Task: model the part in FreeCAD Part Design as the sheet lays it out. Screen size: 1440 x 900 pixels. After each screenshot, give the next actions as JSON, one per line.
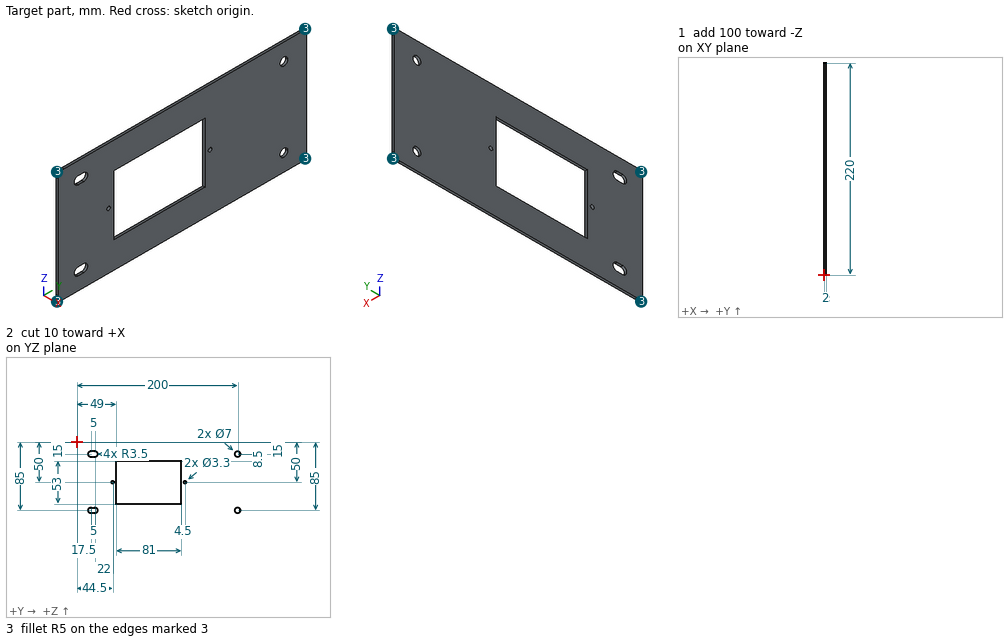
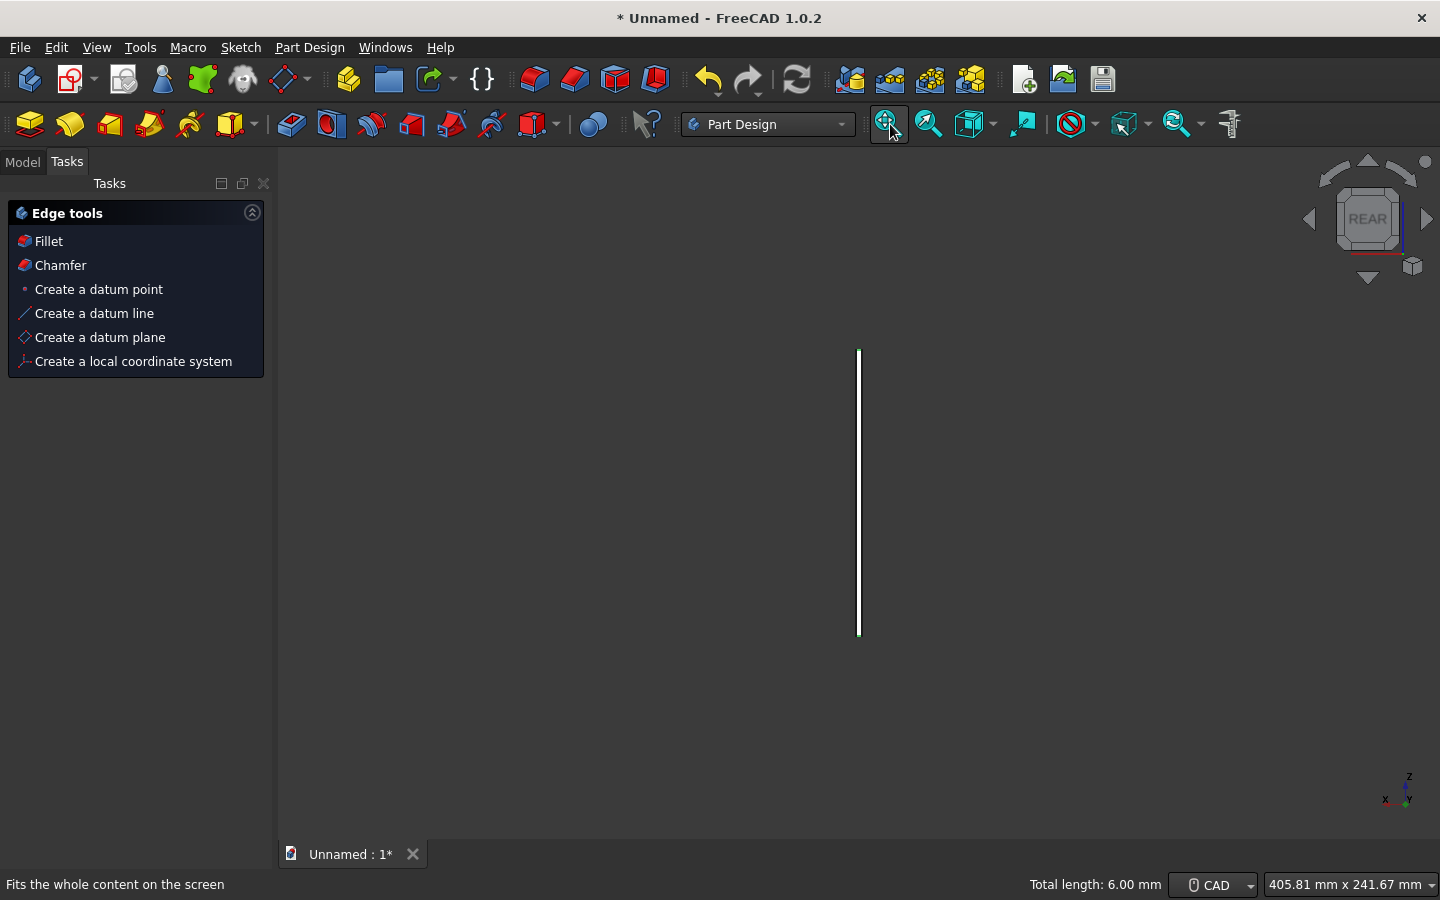
{"action": "key", "text": "6"}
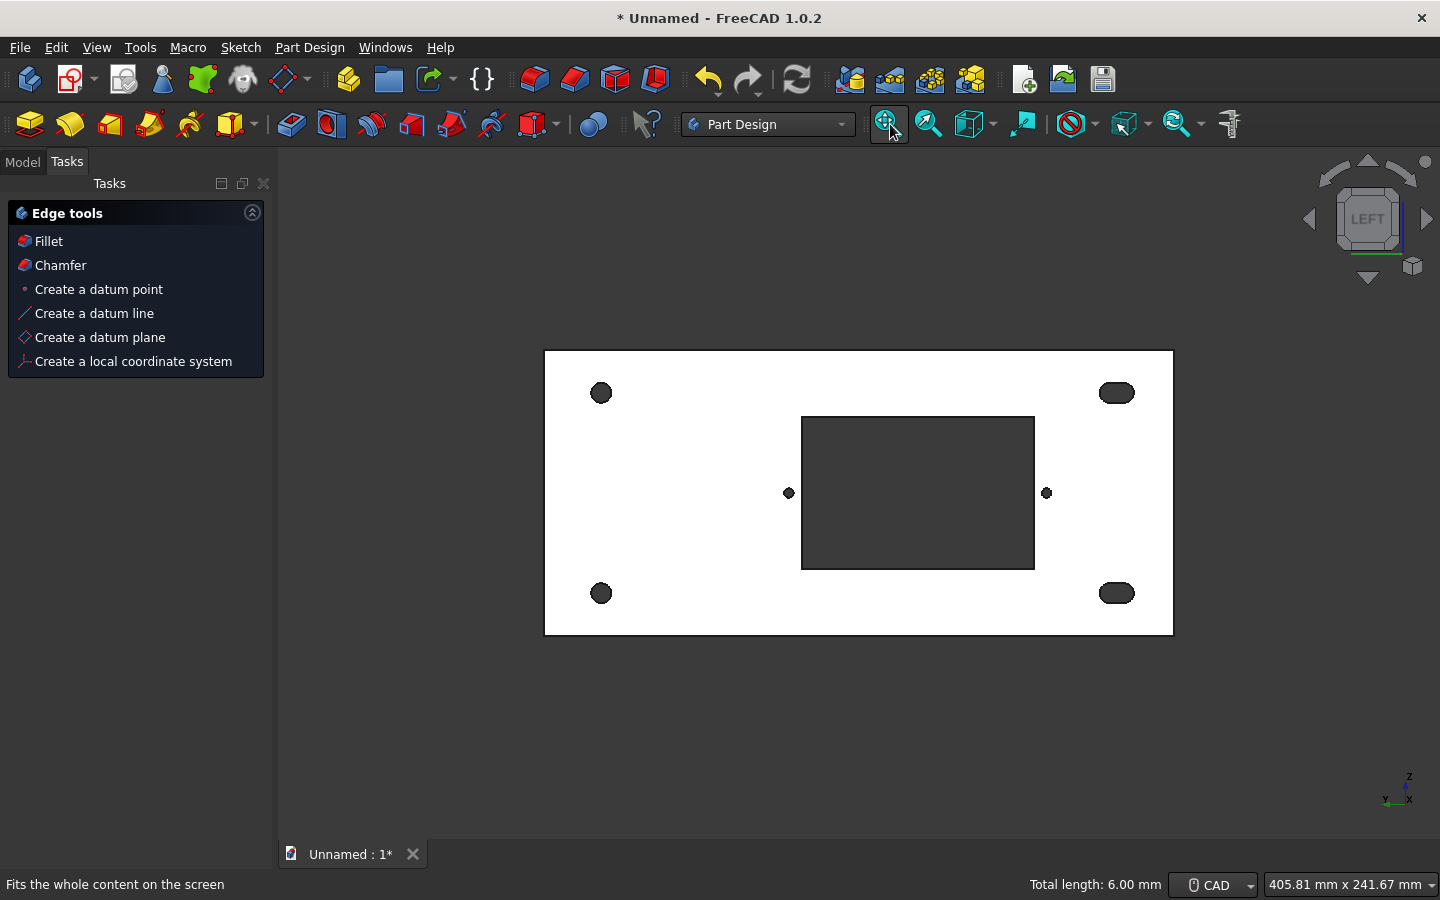
{"action": "scroll", "coordinate": [1174, 349], "scroll_direction": "up", "scroll_amount": 10}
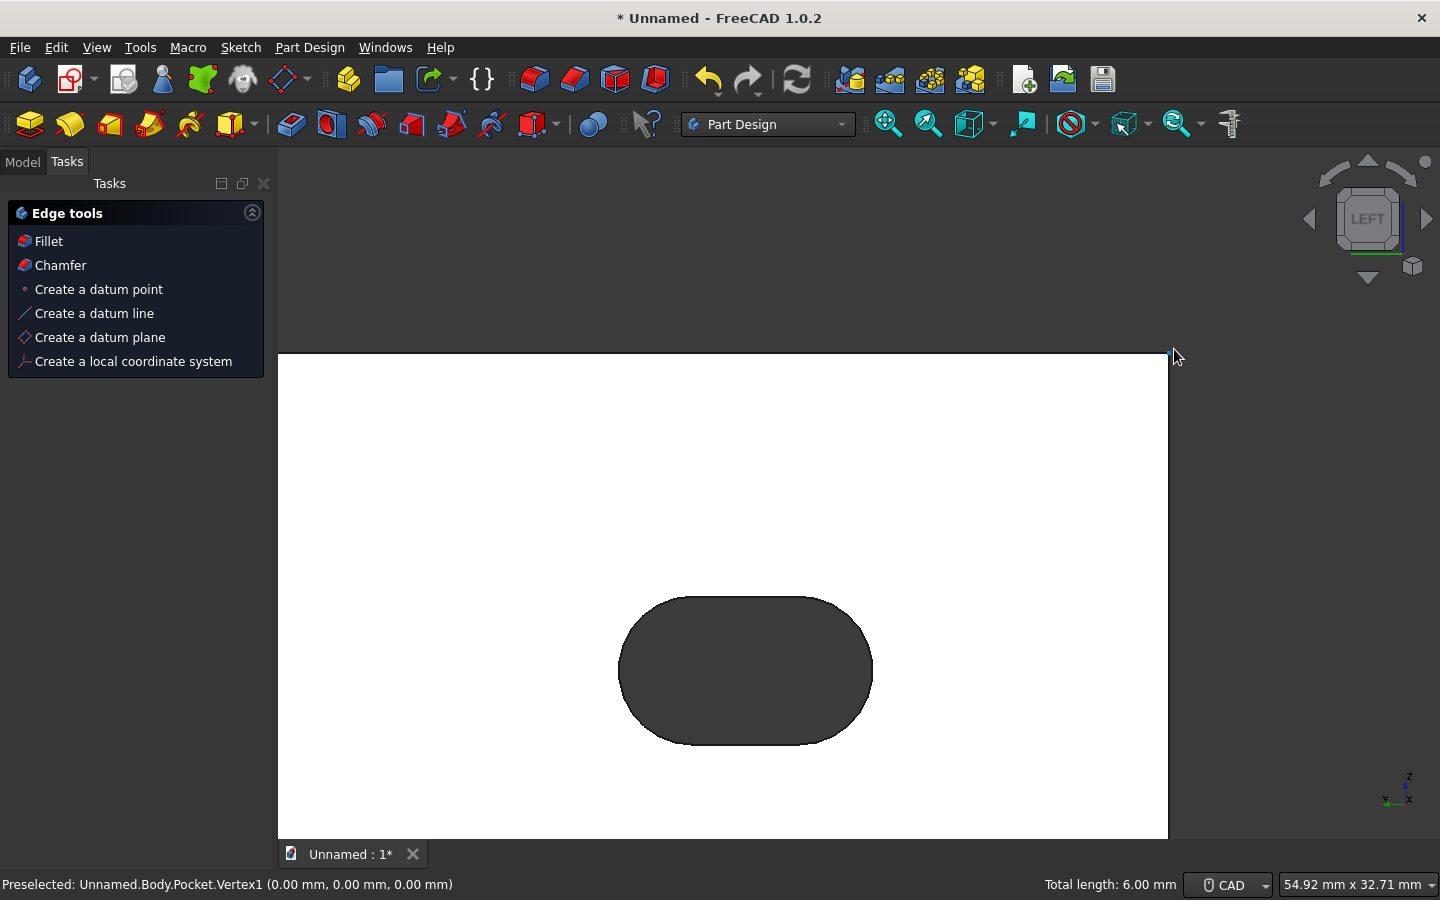
{"action": "left_click", "coordinate": [890, 124]}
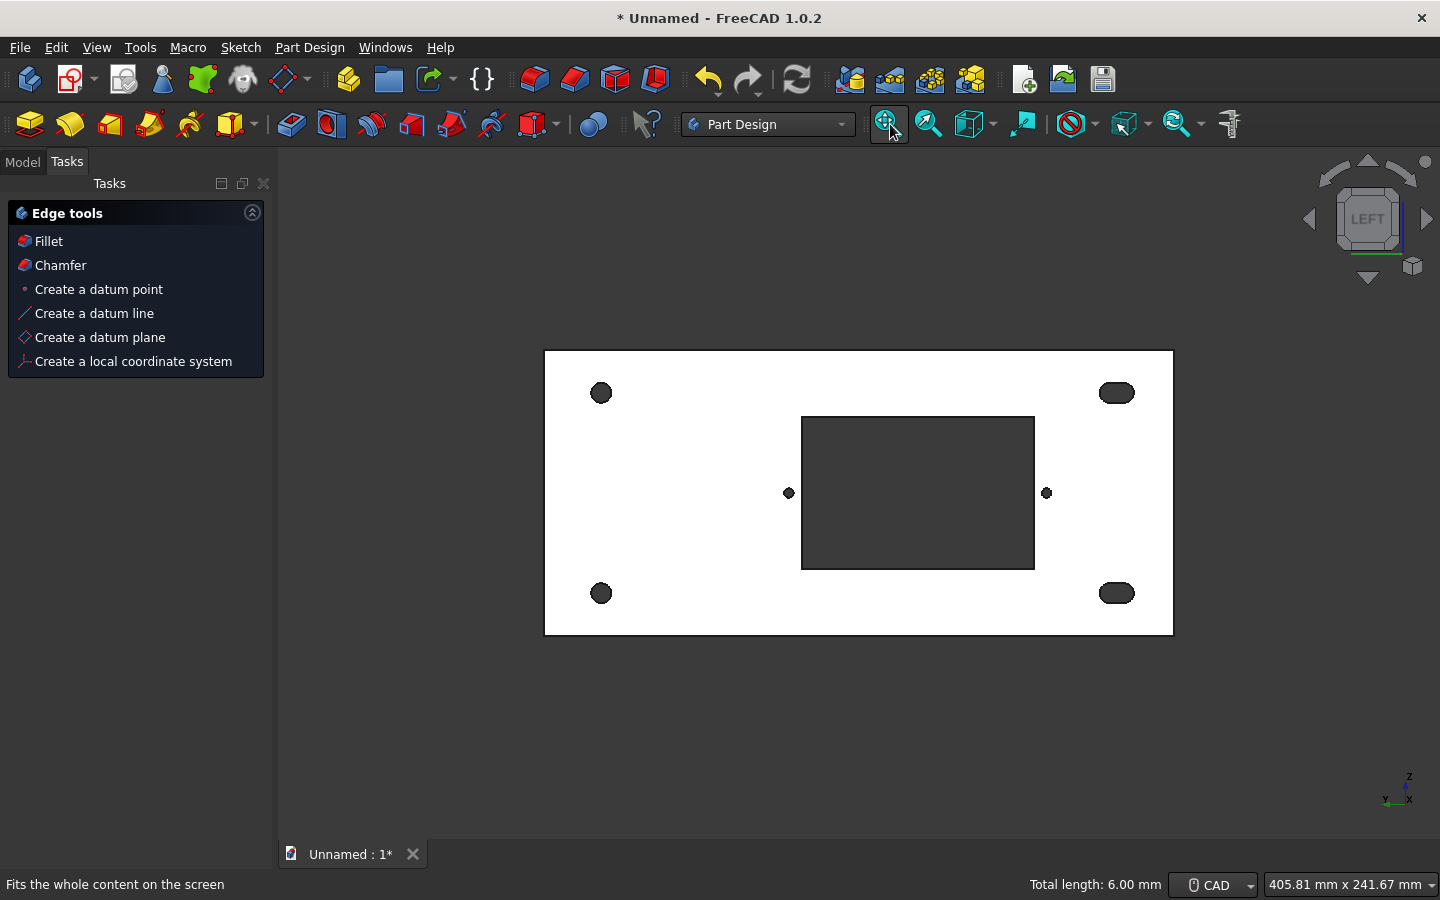
{"action": "key", "text": "v 3"}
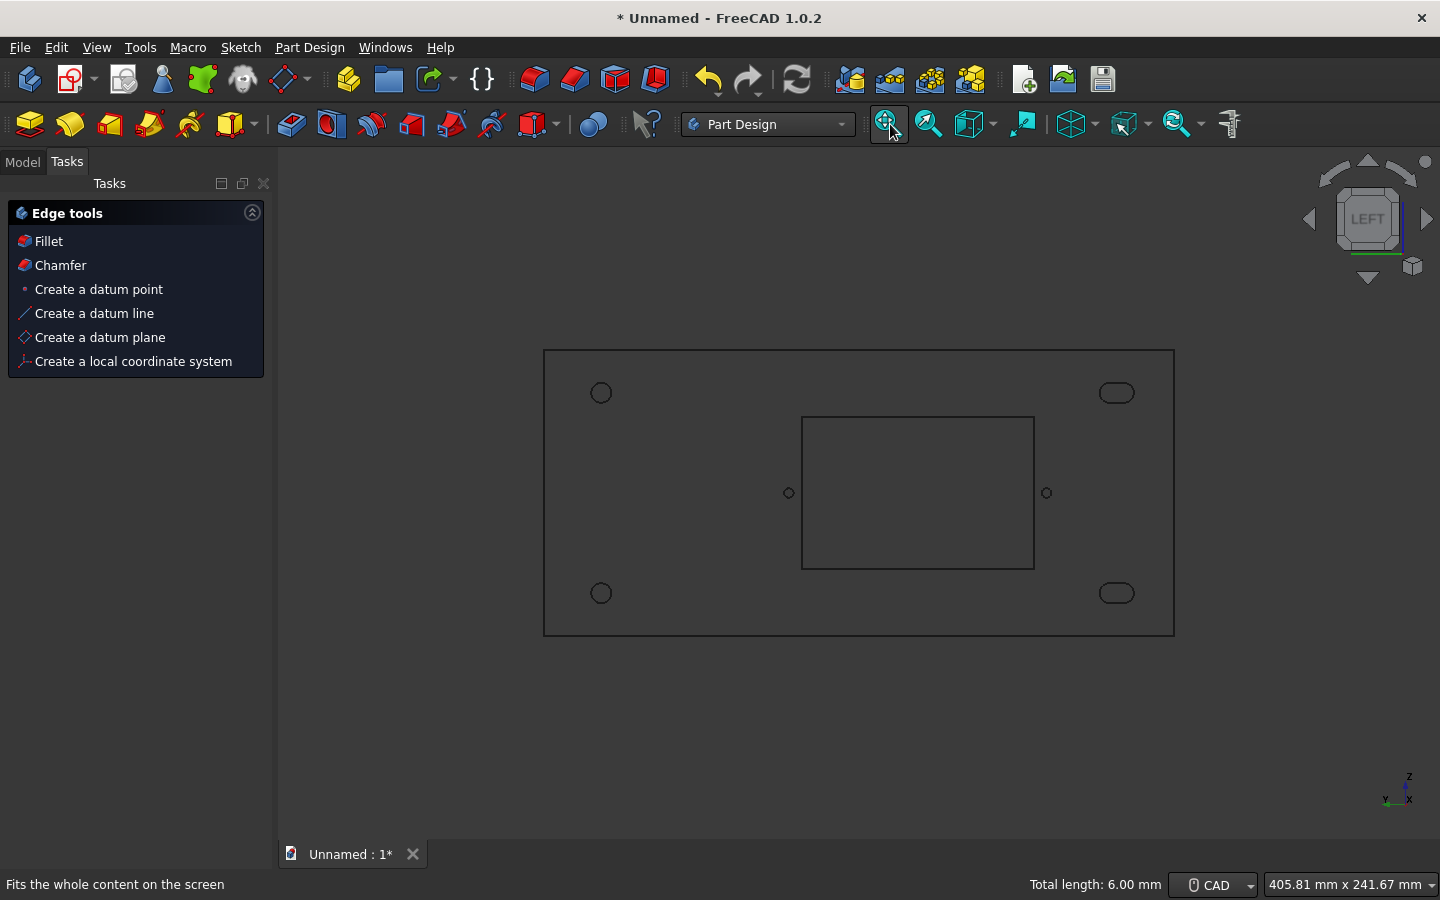
{"action": "key", "text": "0"}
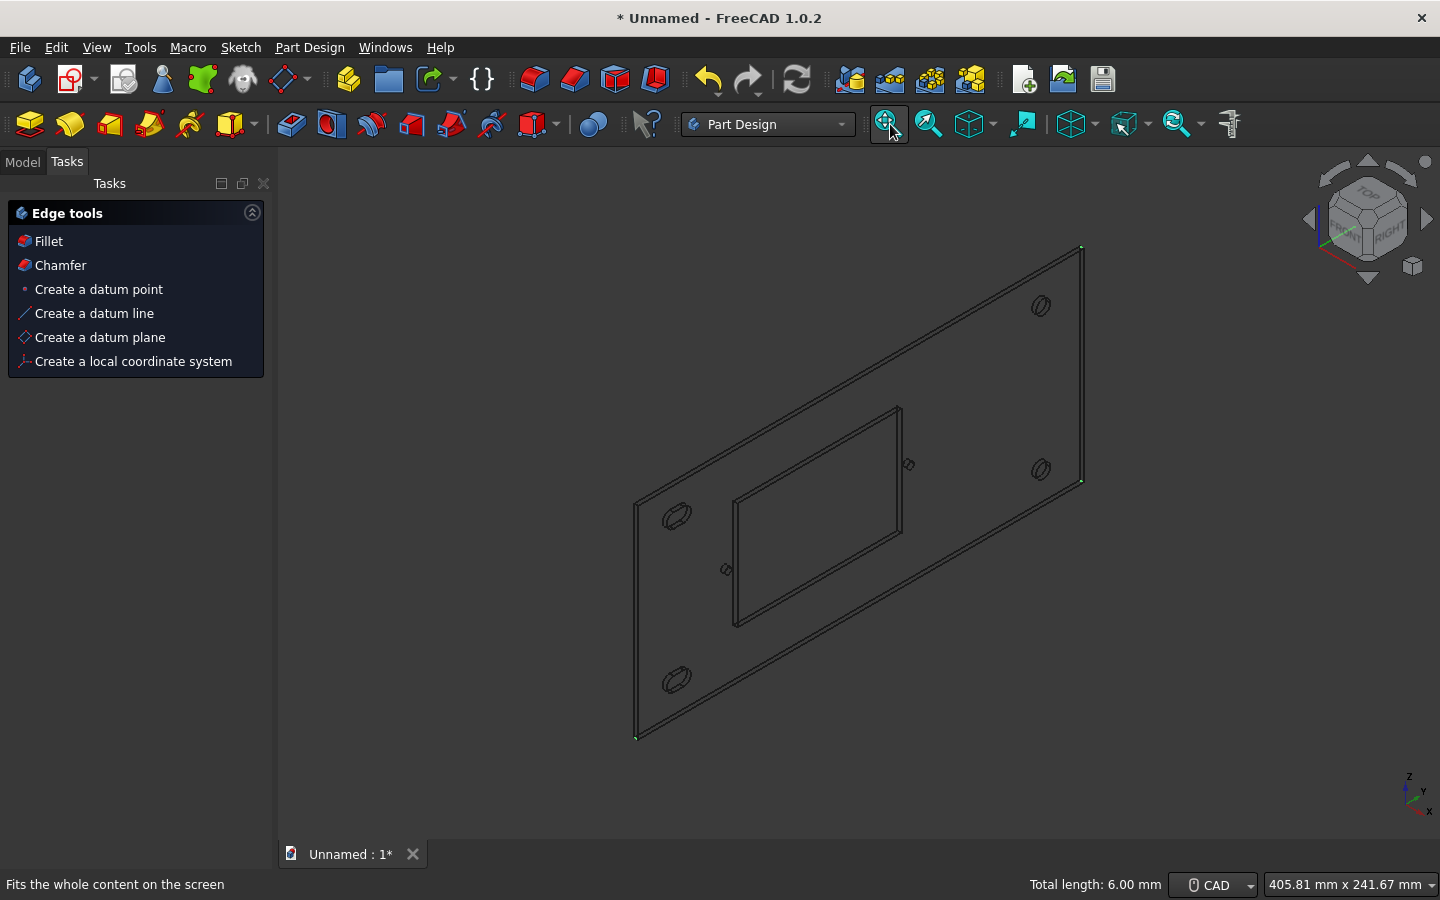
{"action": "scroll", "coordinate": [636, 504], "scroll_direction": "up", "scroll_amount": 10}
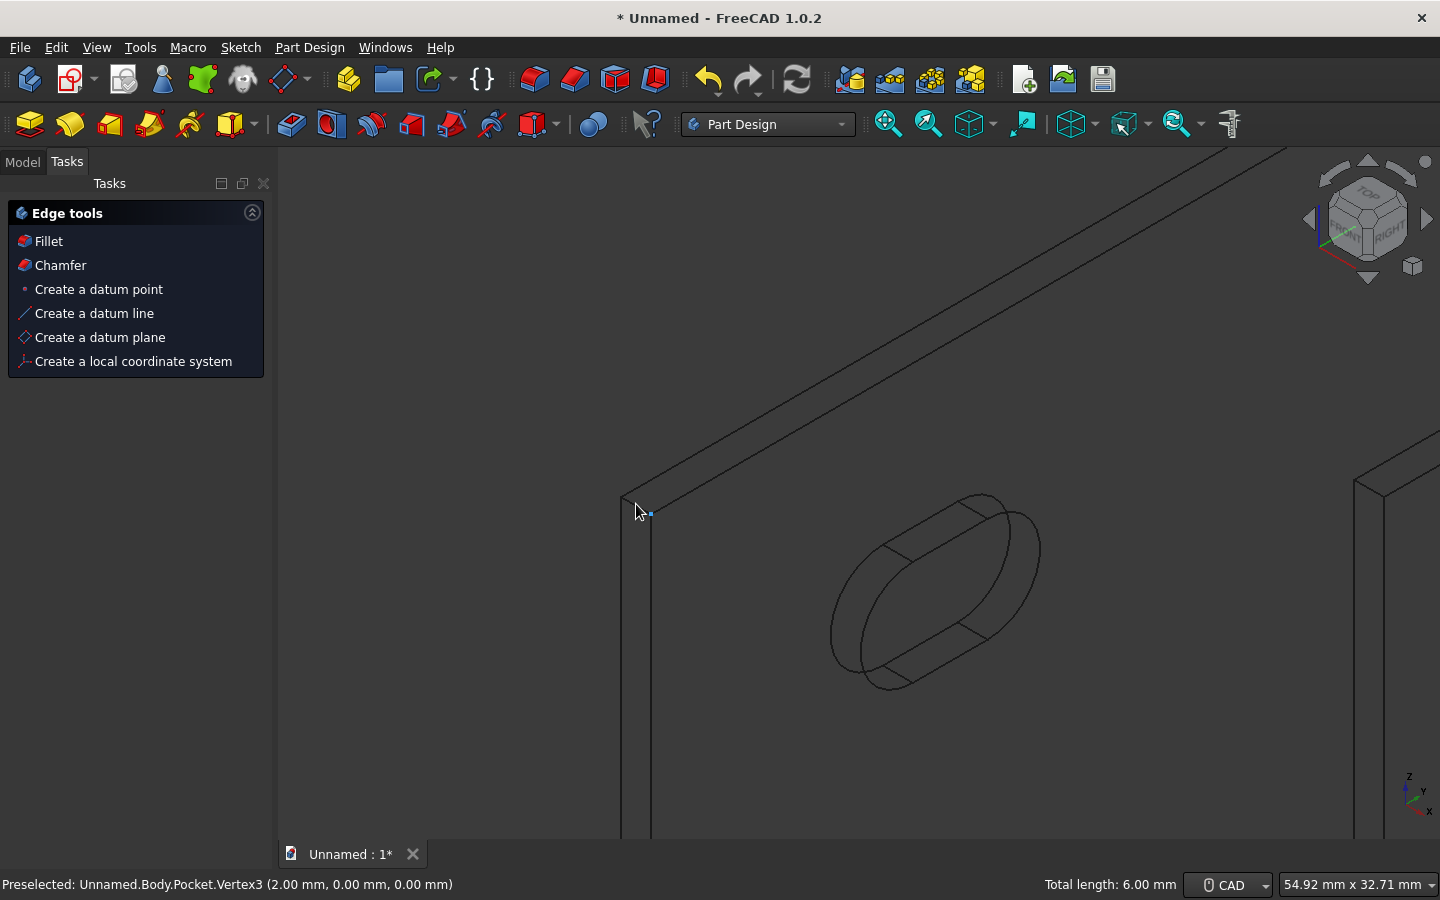
{"action": "left_click", "coordinate": [636, 505], "text": "ctrl"}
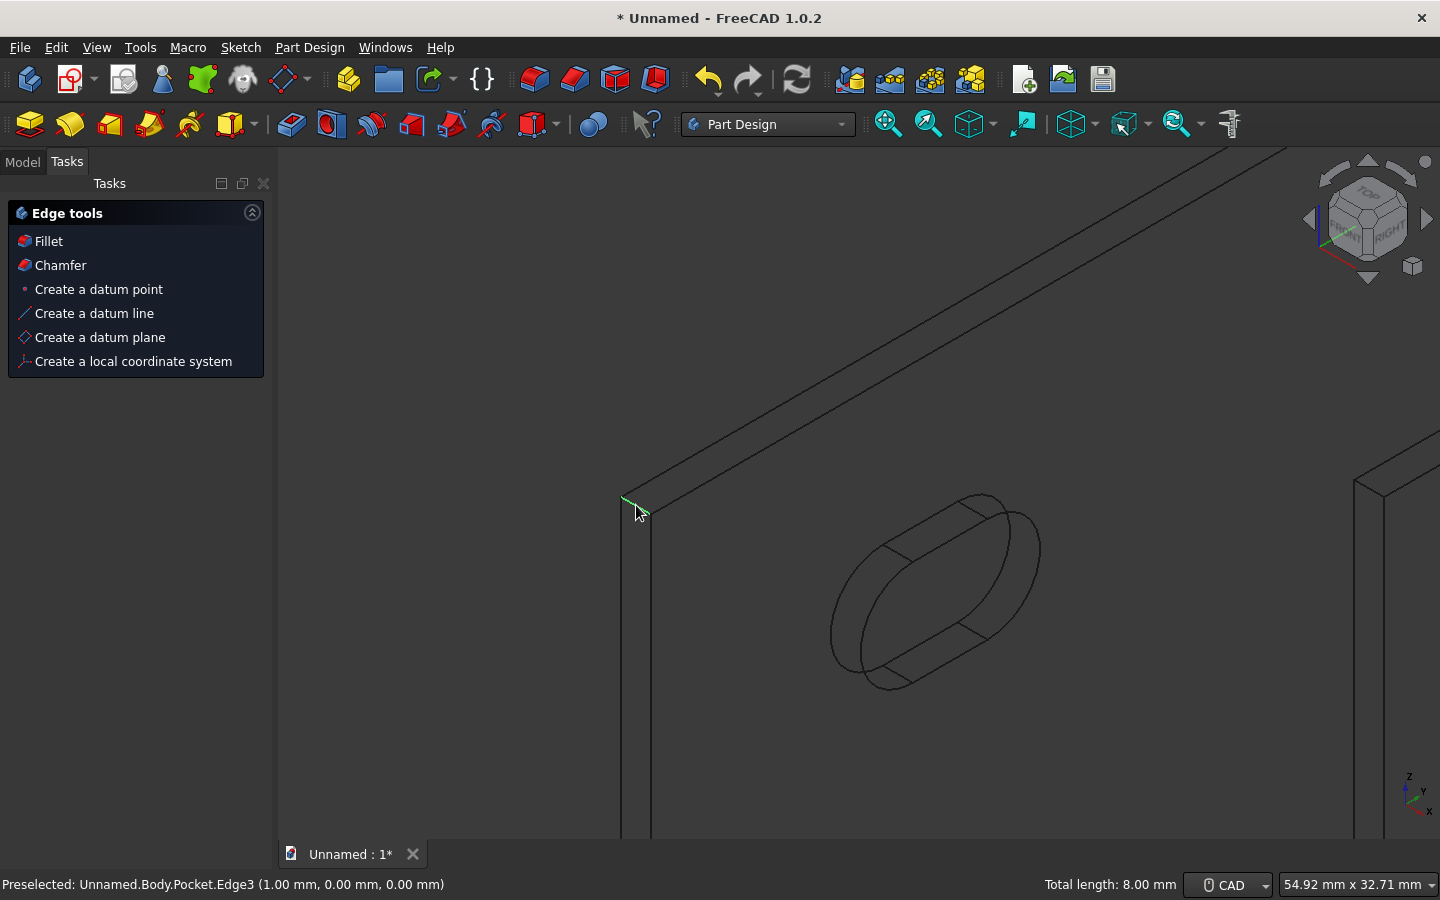
{"action": "key", "text": "v 1"}